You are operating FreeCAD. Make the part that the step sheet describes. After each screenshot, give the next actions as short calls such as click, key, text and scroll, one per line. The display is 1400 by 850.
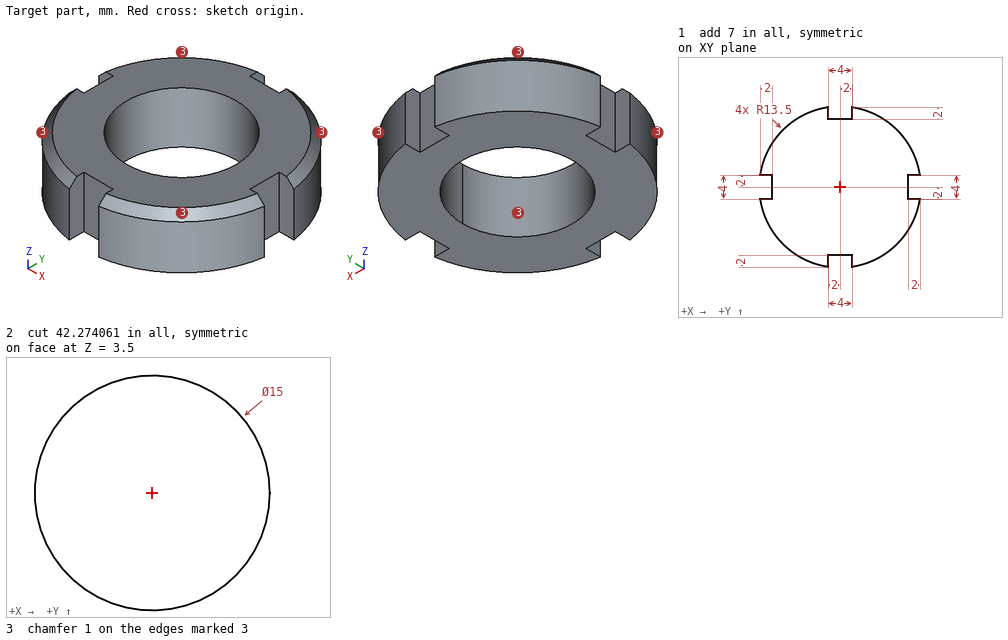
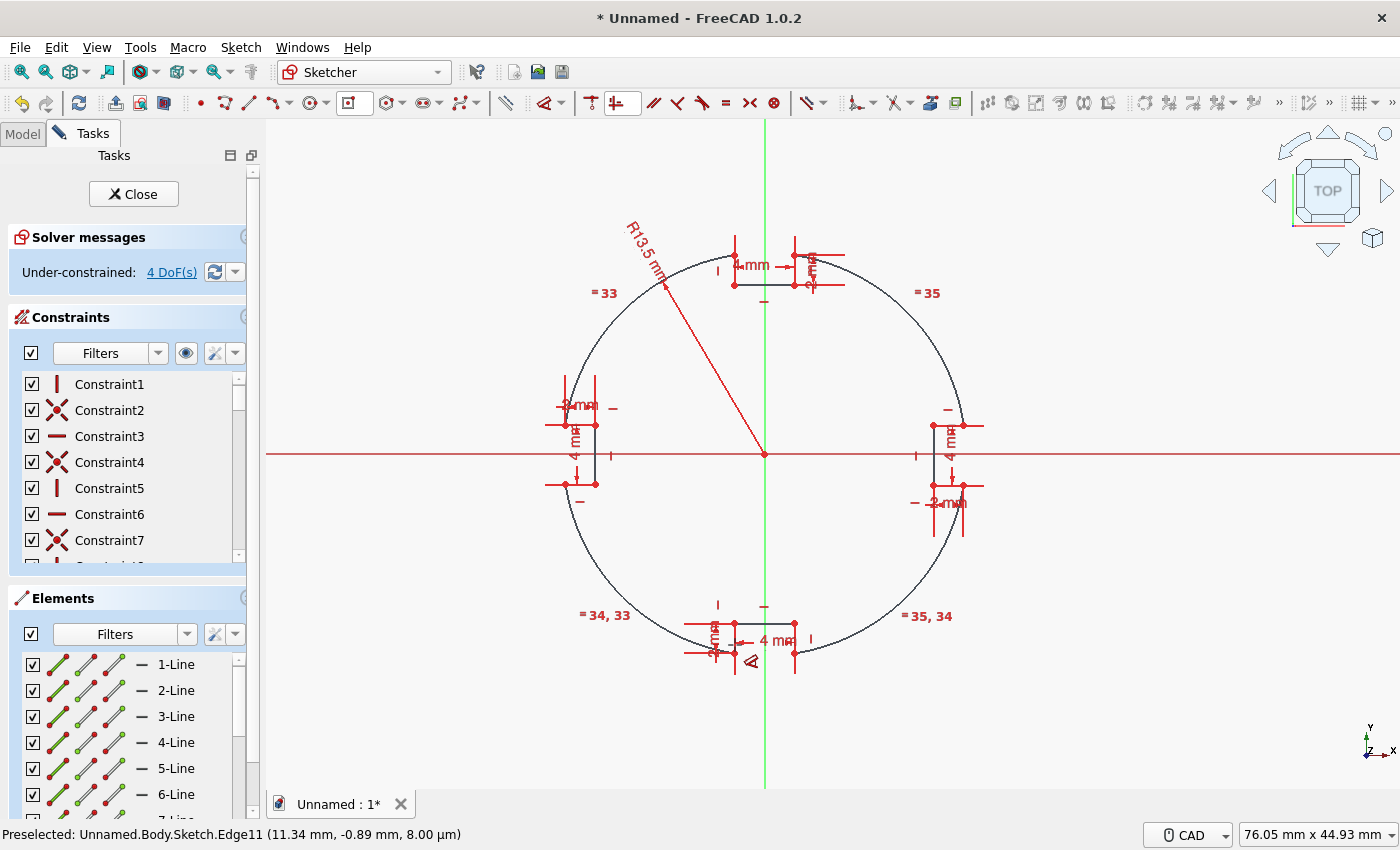
scroll(795, 255, up, 2)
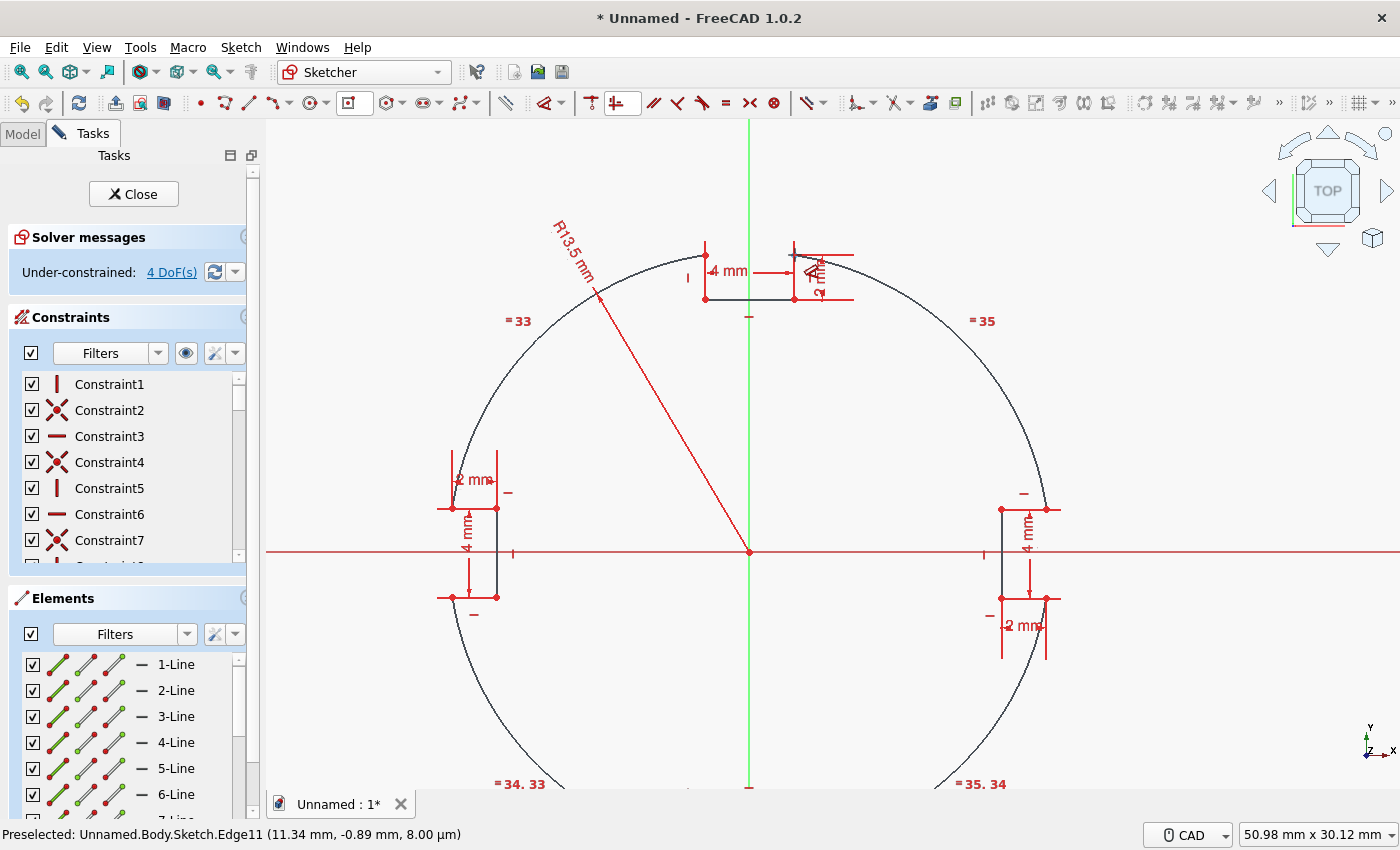
click(794, 255)
click(772, 221)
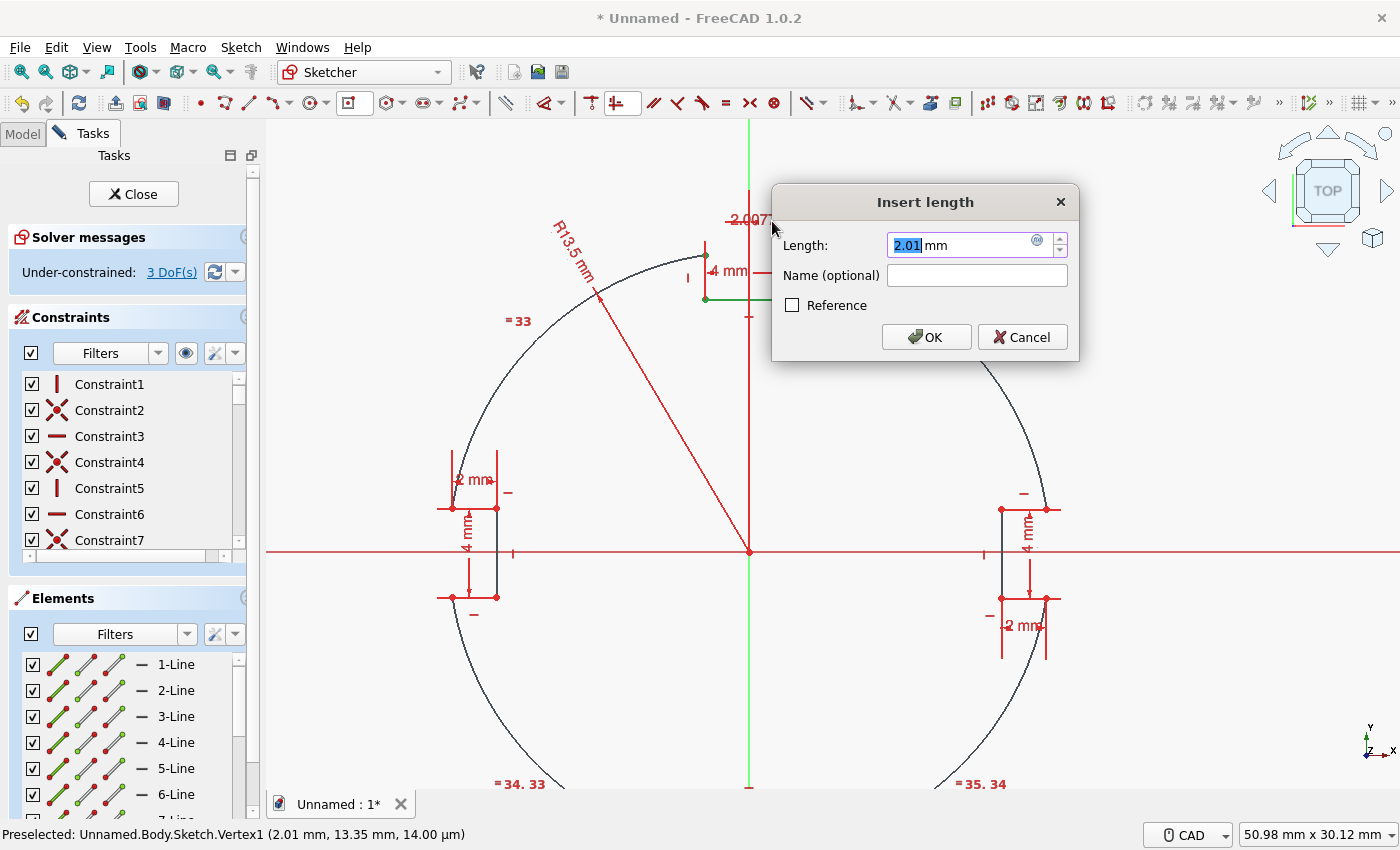
text(2)
key(Return)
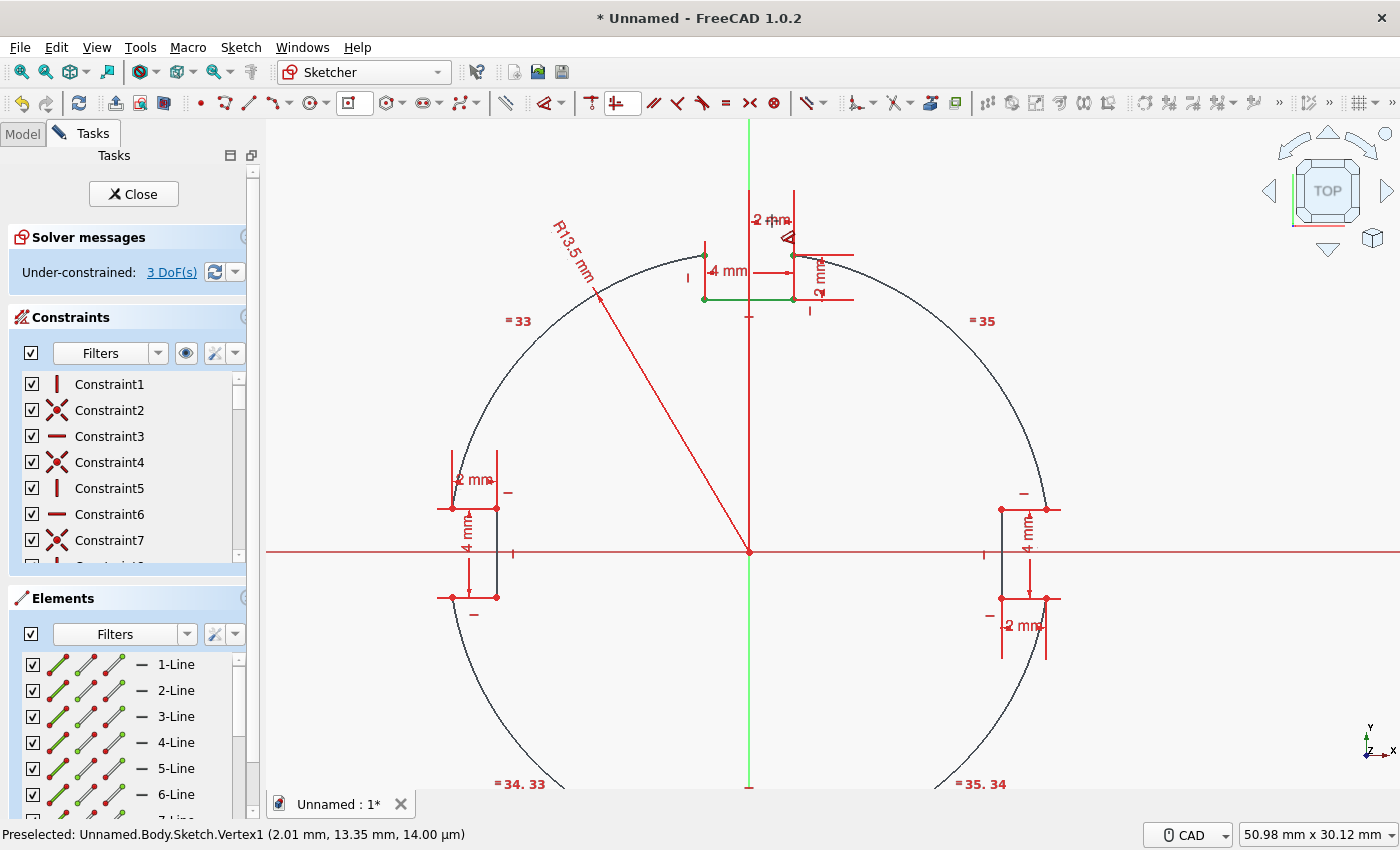
click(452, 509)
click(783, 531)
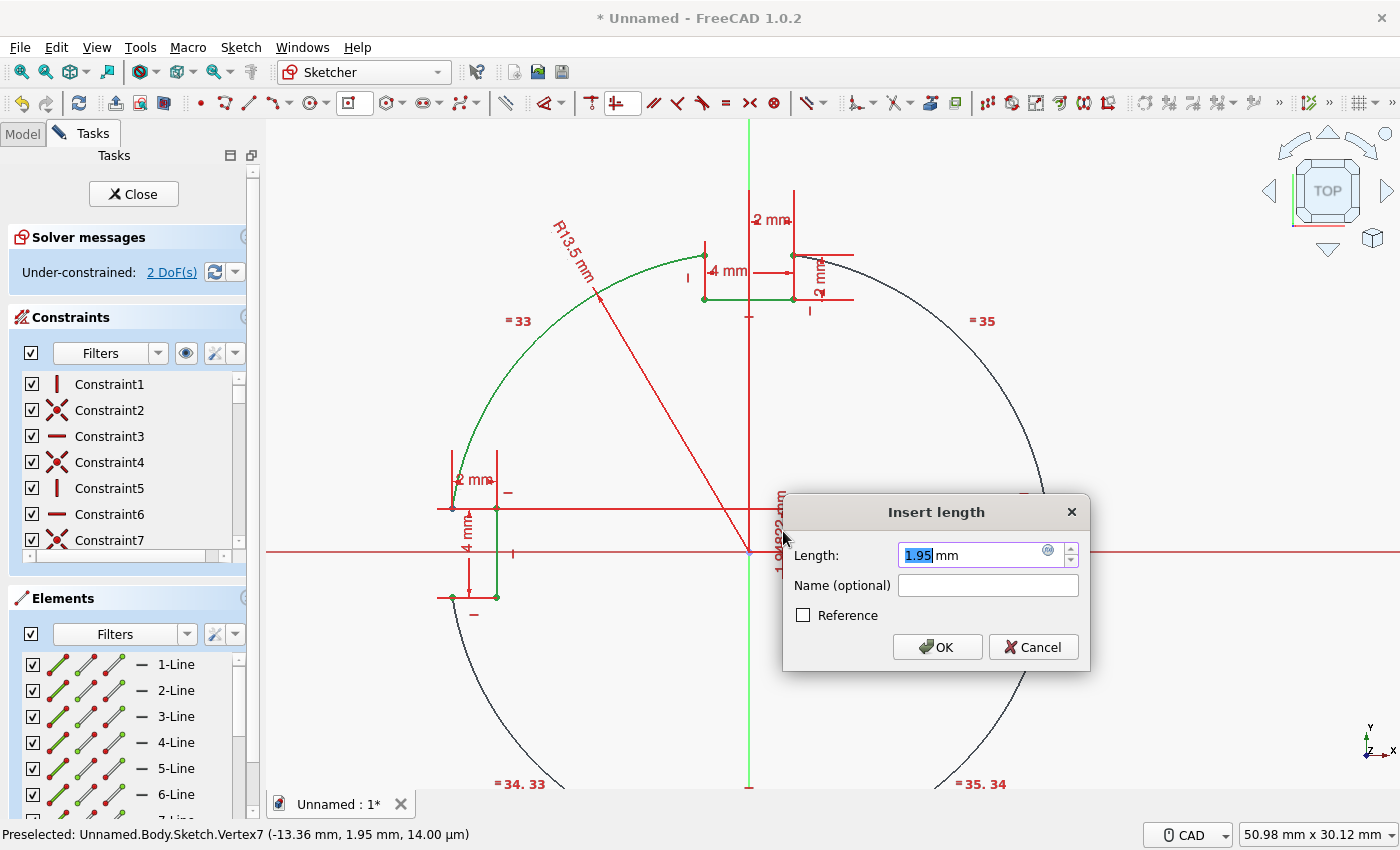
text(2)
key(Return)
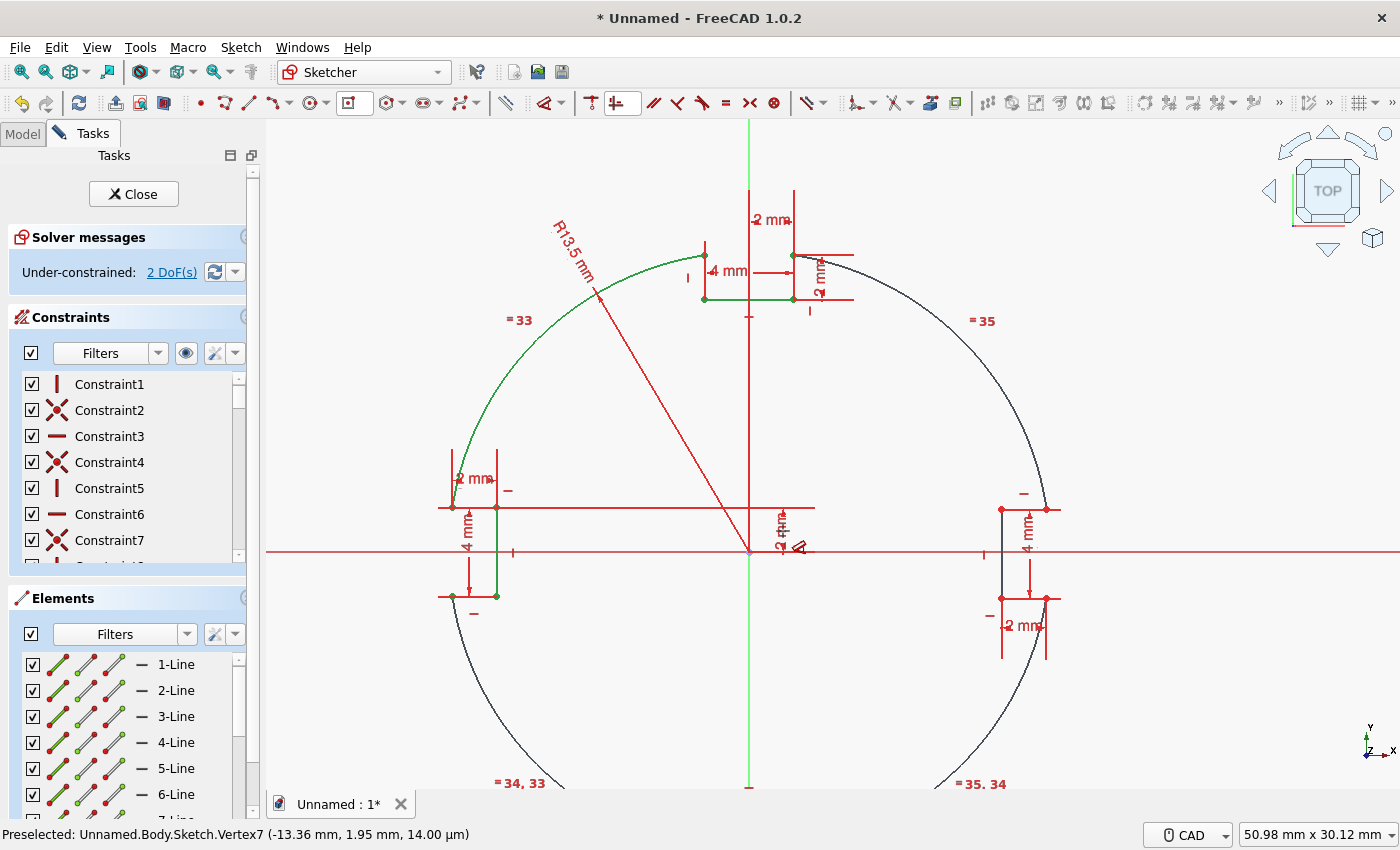
scroll(795, 254, down, 2)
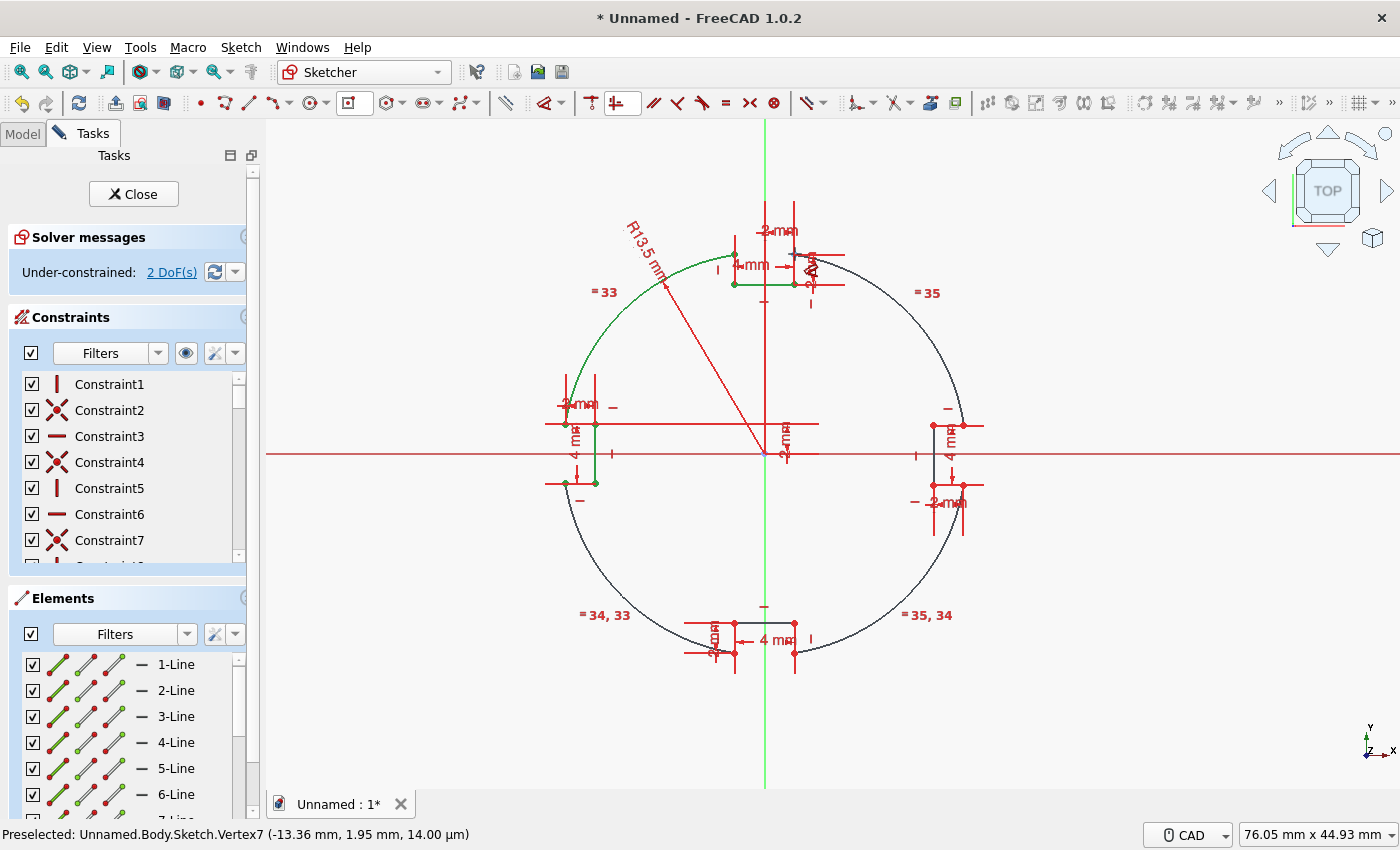
scroll(735, 653, up, 2)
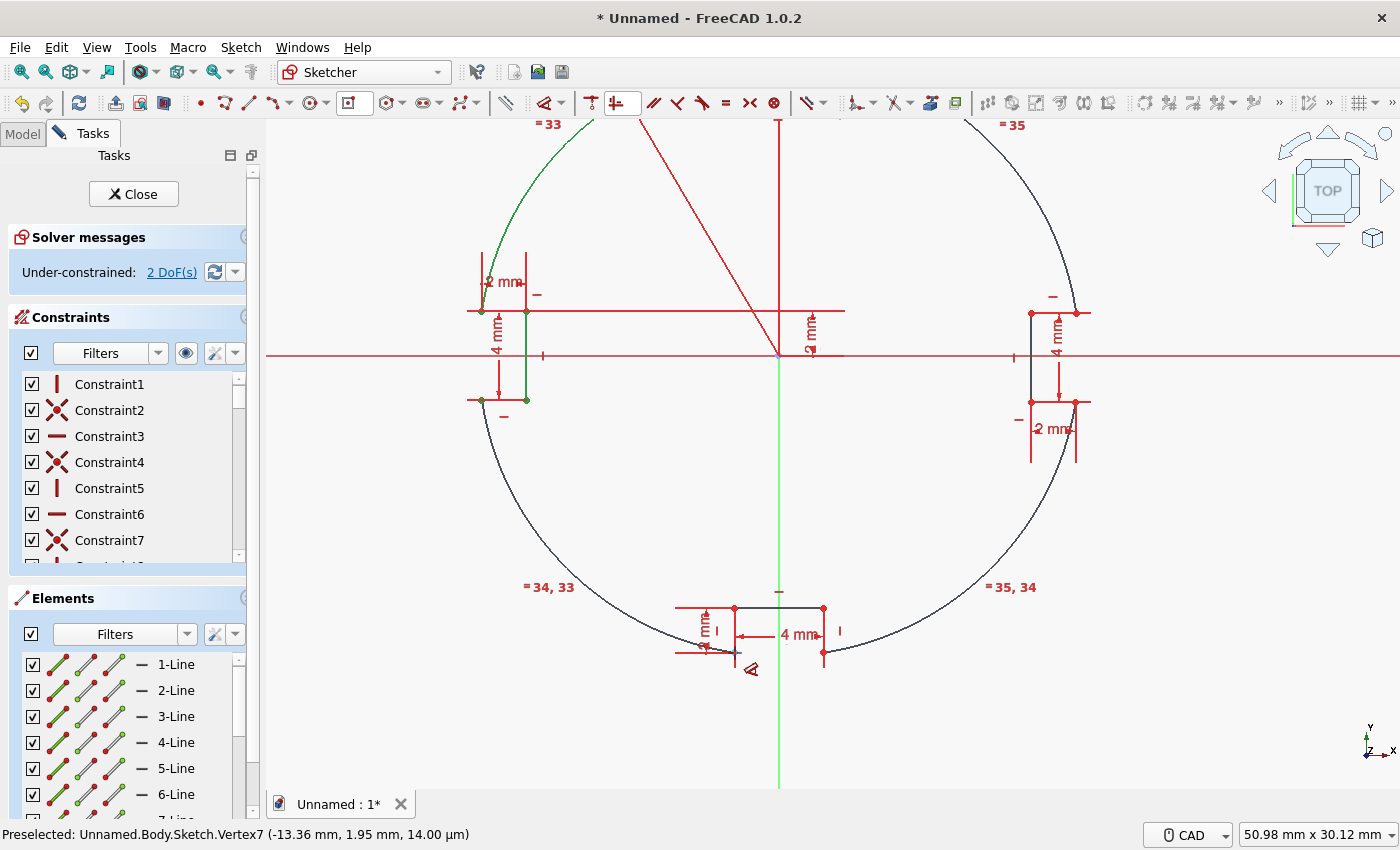
click(735, 653)
click(757, 687)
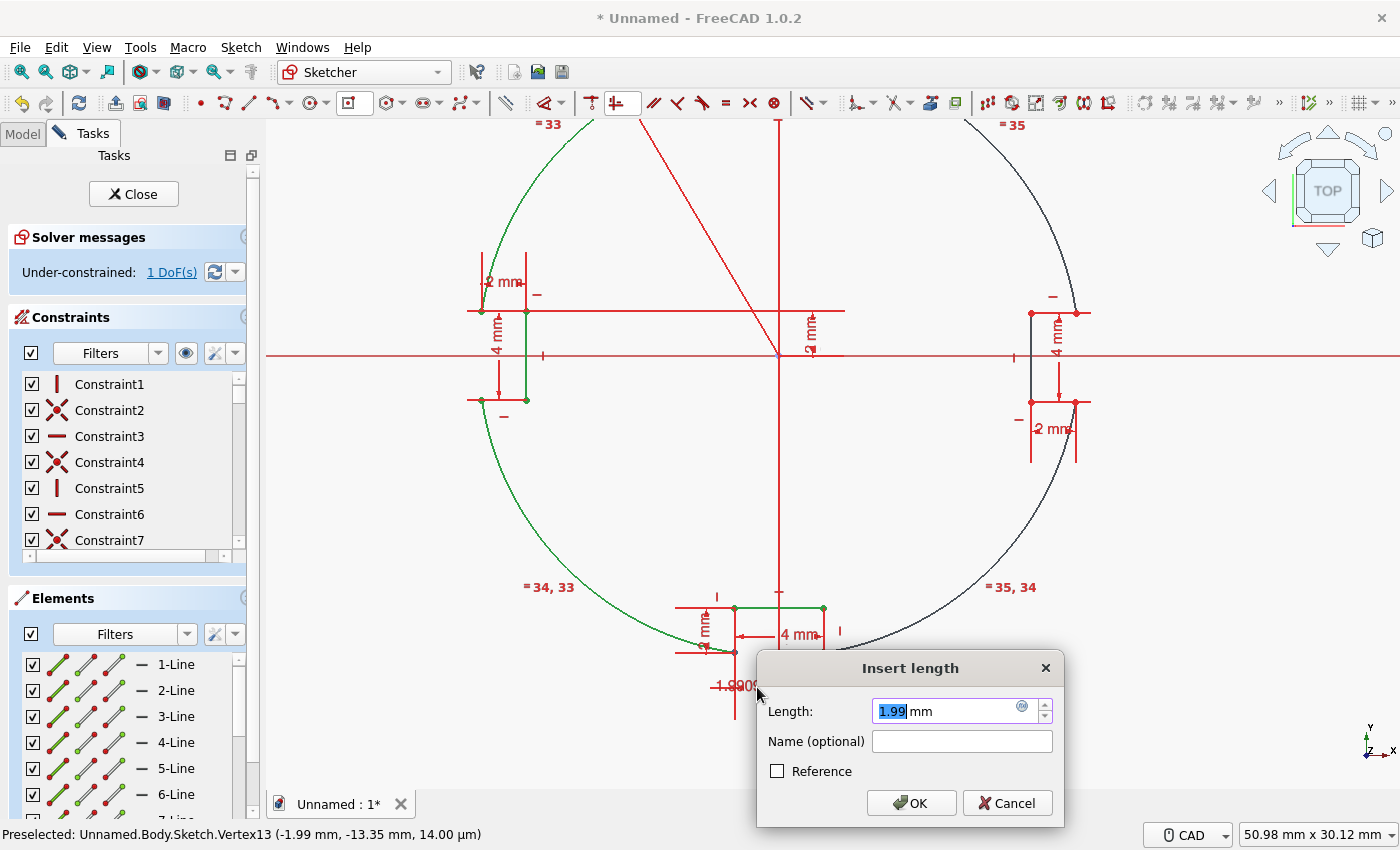
text(2)
key(Return)